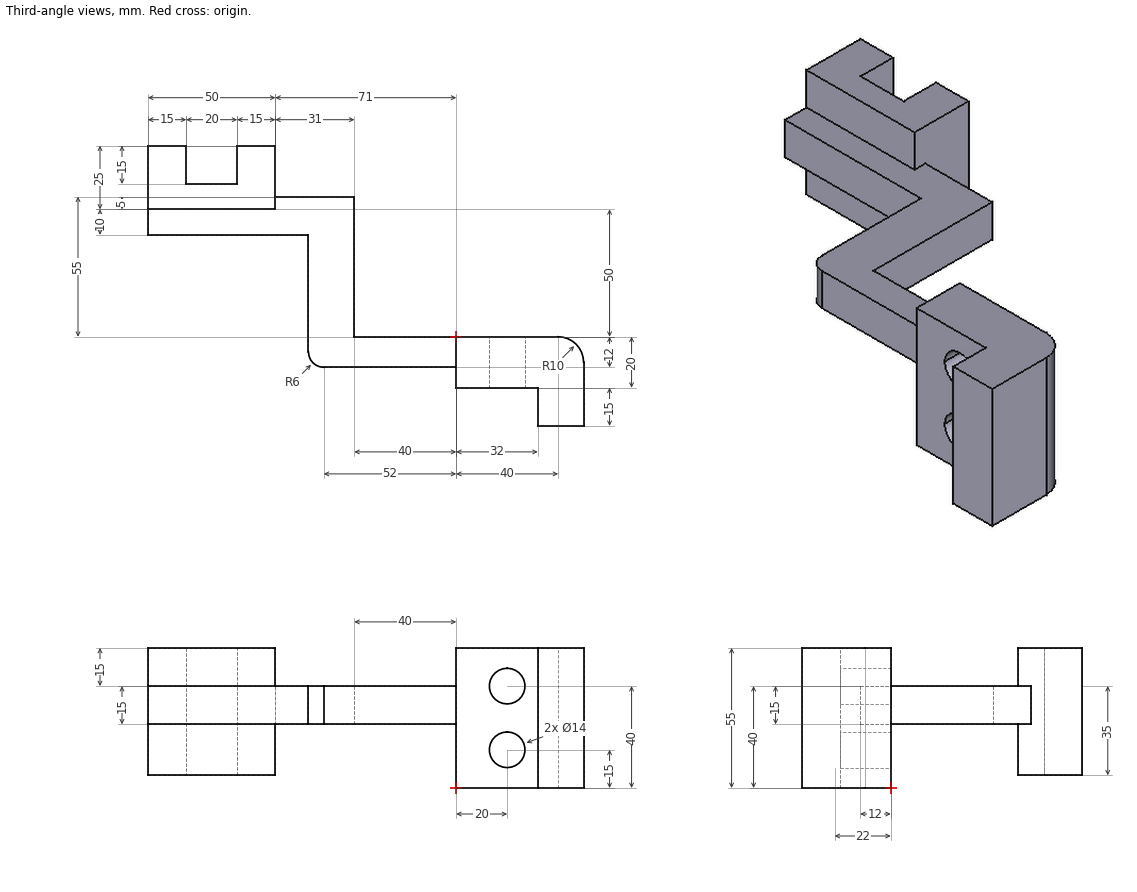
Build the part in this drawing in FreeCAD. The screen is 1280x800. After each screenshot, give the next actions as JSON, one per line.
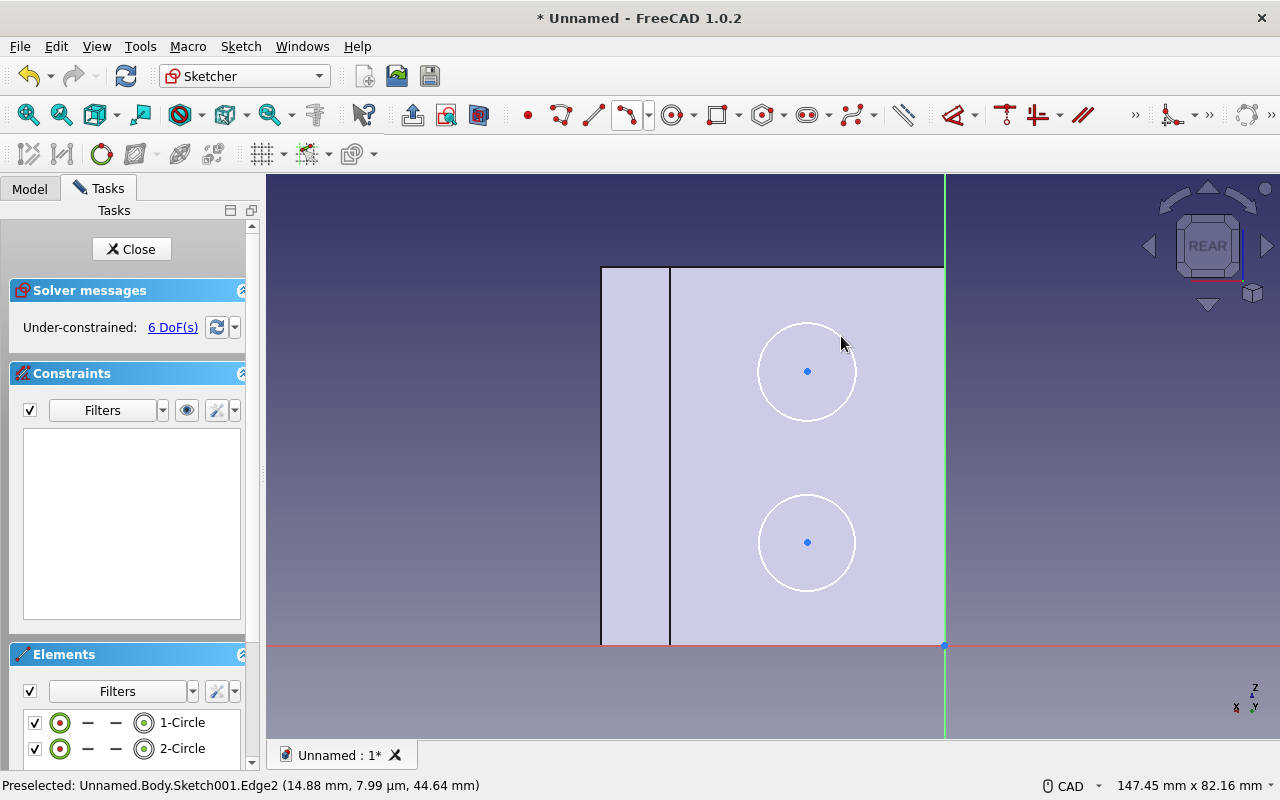
{"action": "left_click", "coordinate": [841, 509]}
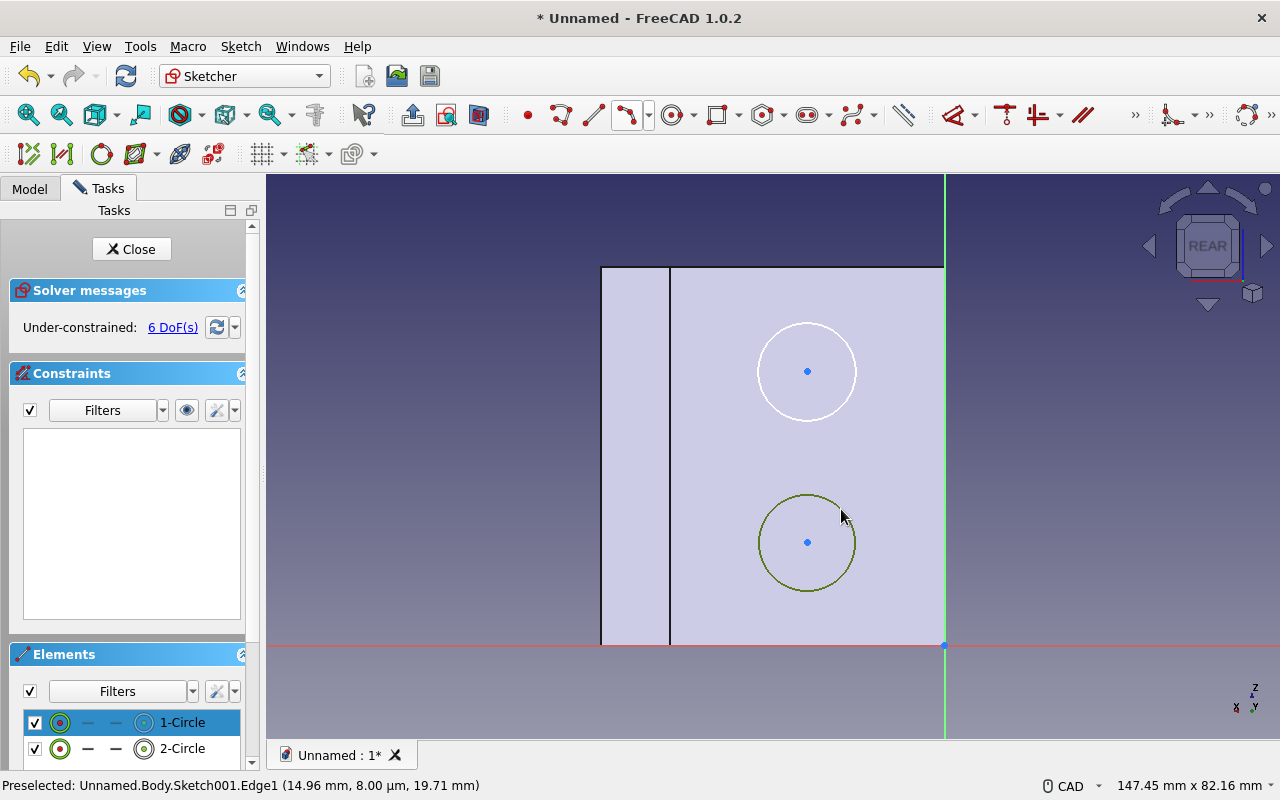
{"action": "left_click", "coordinate": [841, 337]}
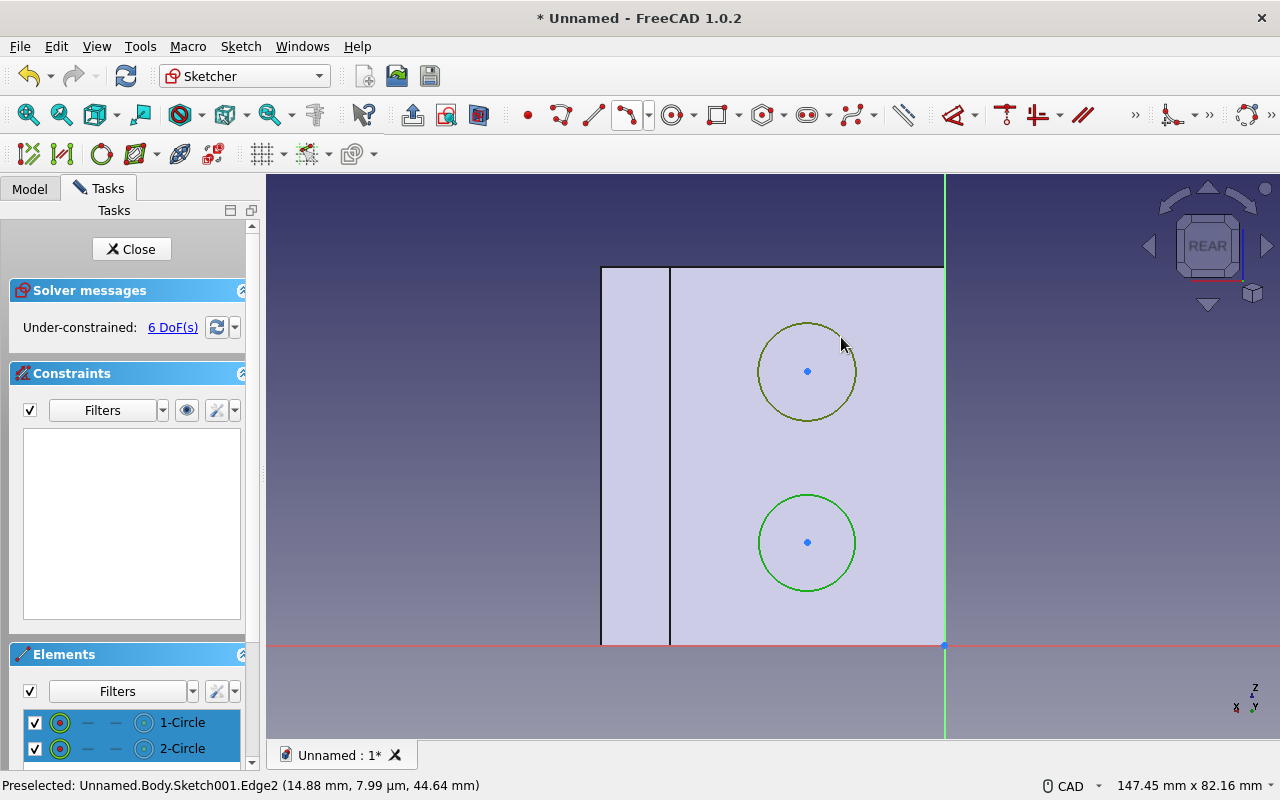
{"action": "key", "text": "e"}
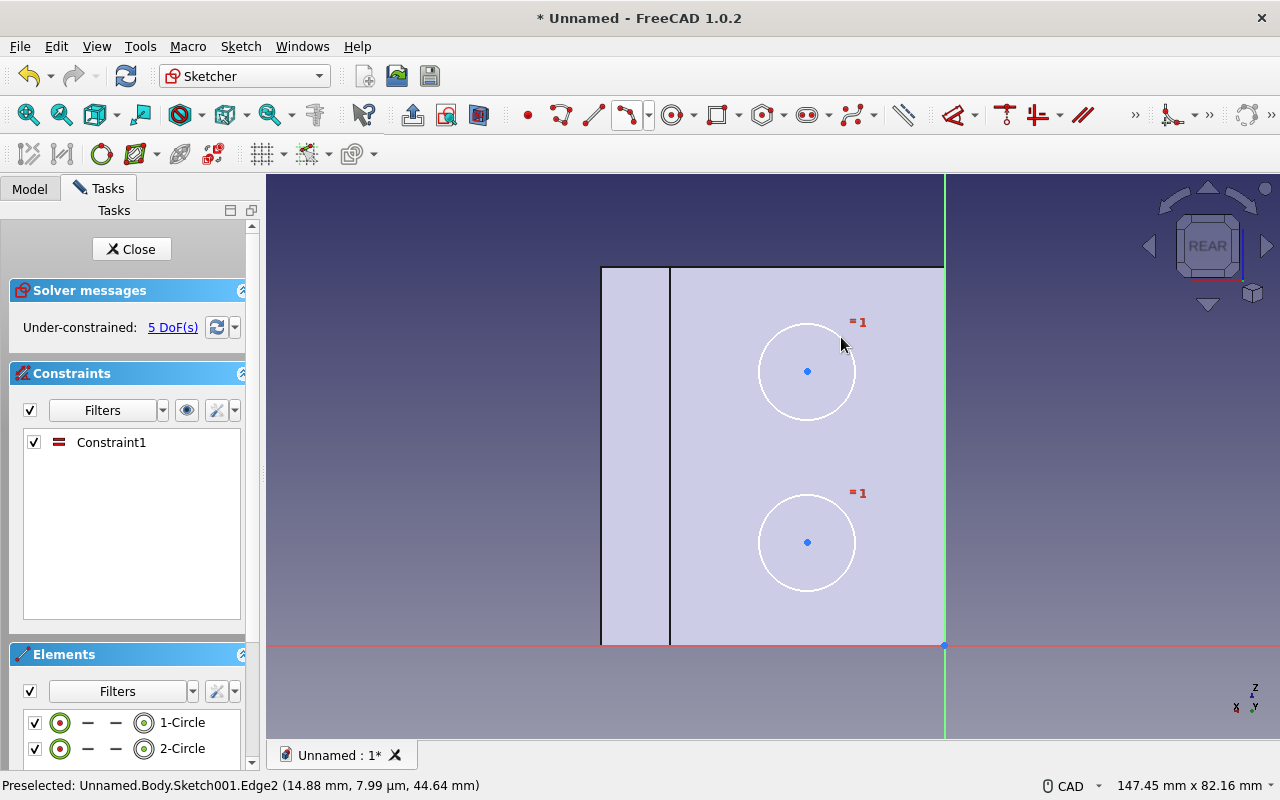
{"action": "left_click", "coordinate": [807, 543]}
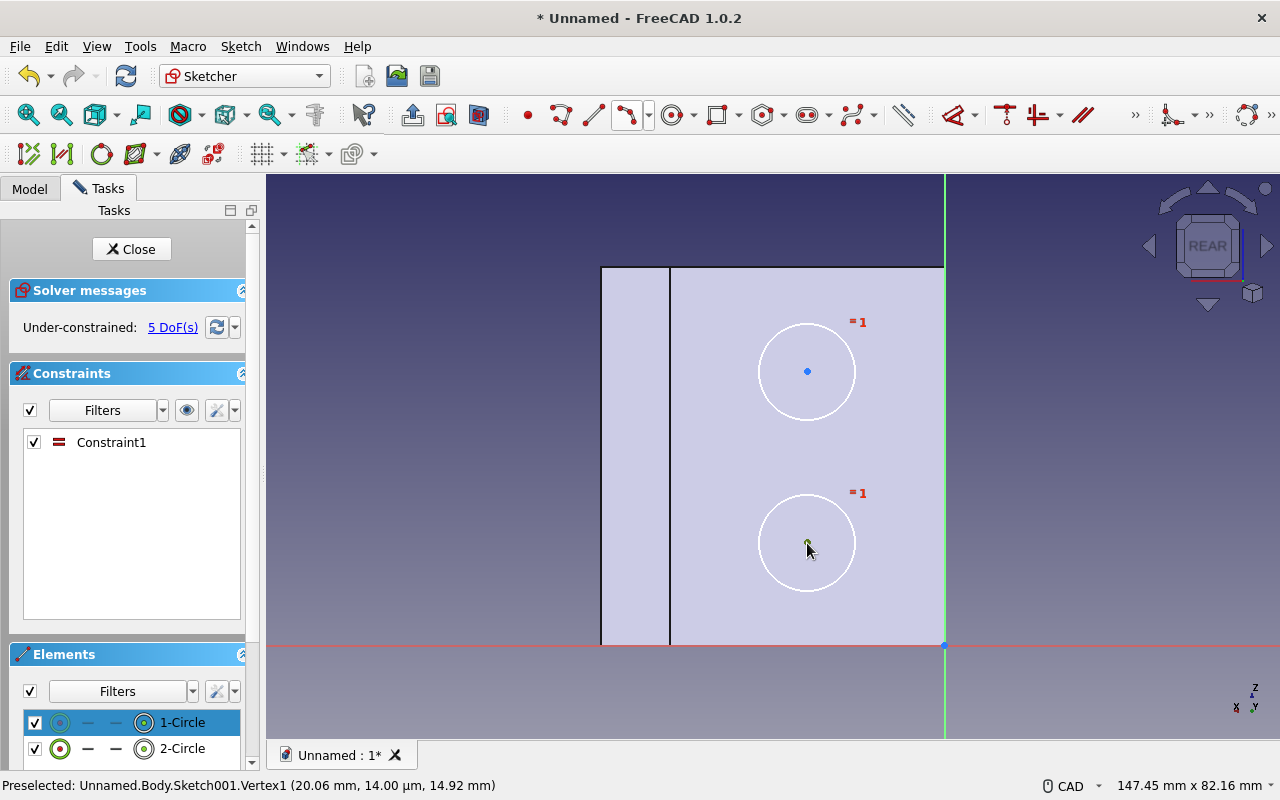
{"action": "left_click", "coordinate": [807, 372]}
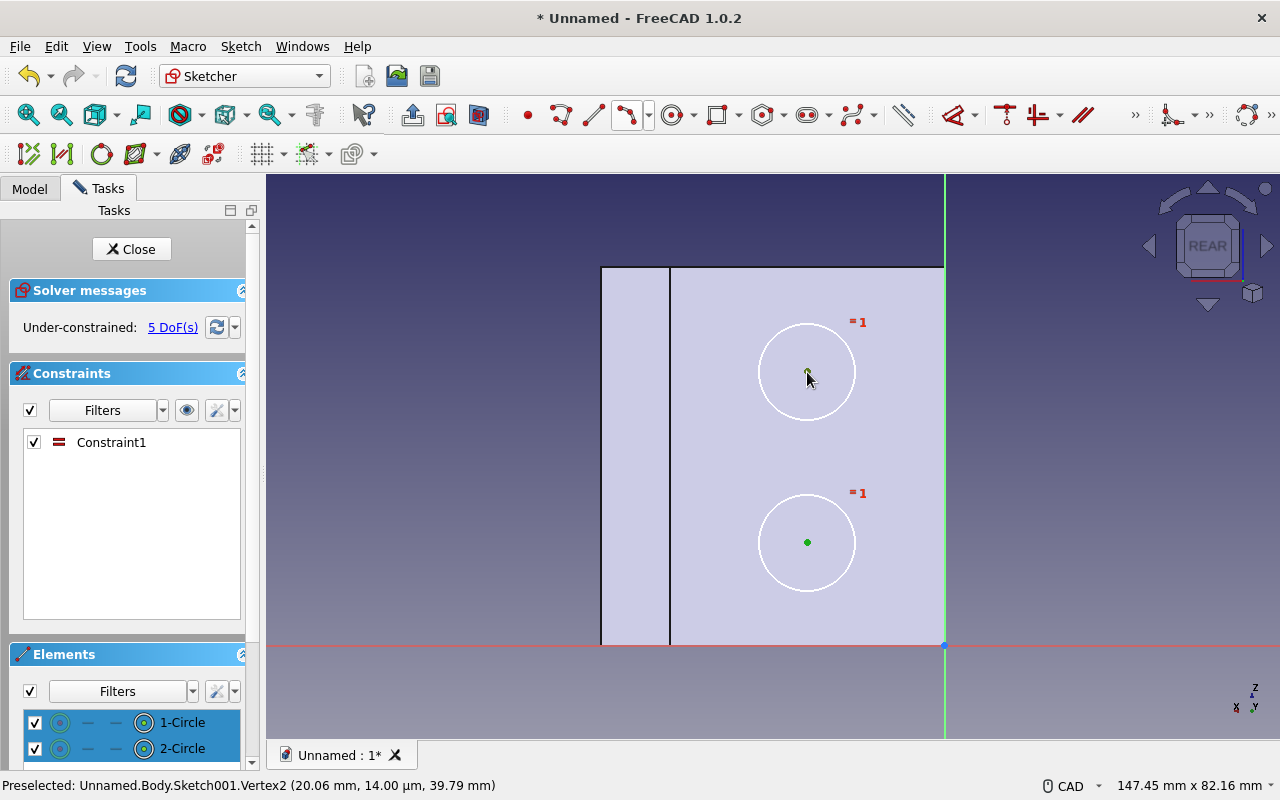
{"action": "left_click", "coordinate": [1060, 116]}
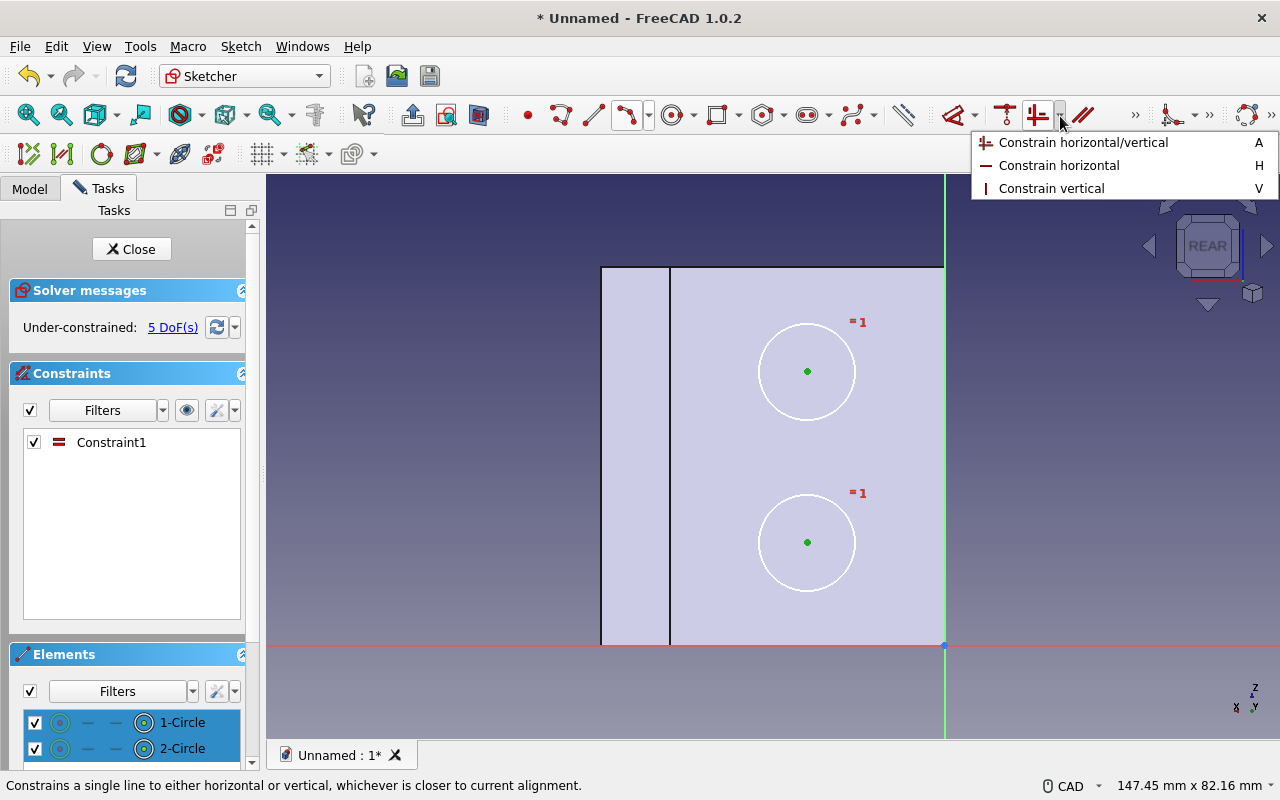
{"action": "left_click", "coordinate": [1125, 188]}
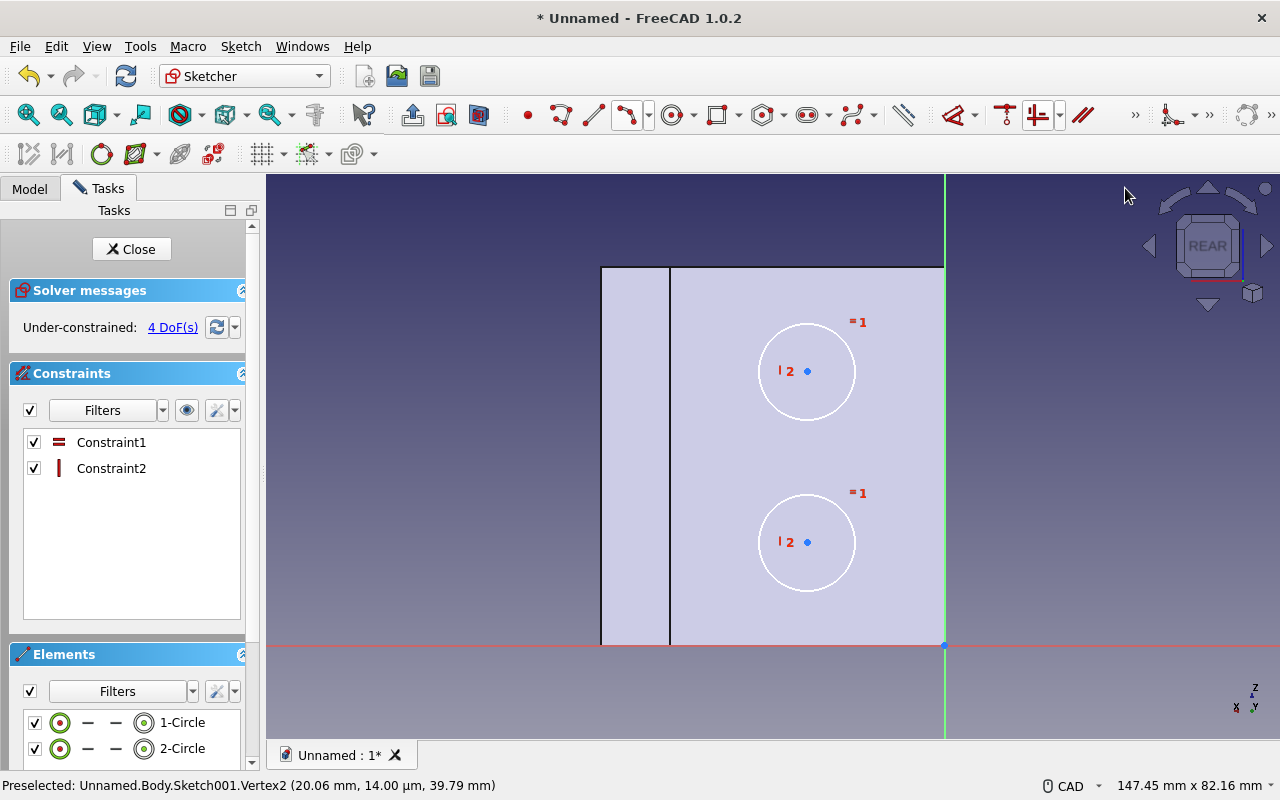
{"action": "left_click", "coordinate": [952, 116]}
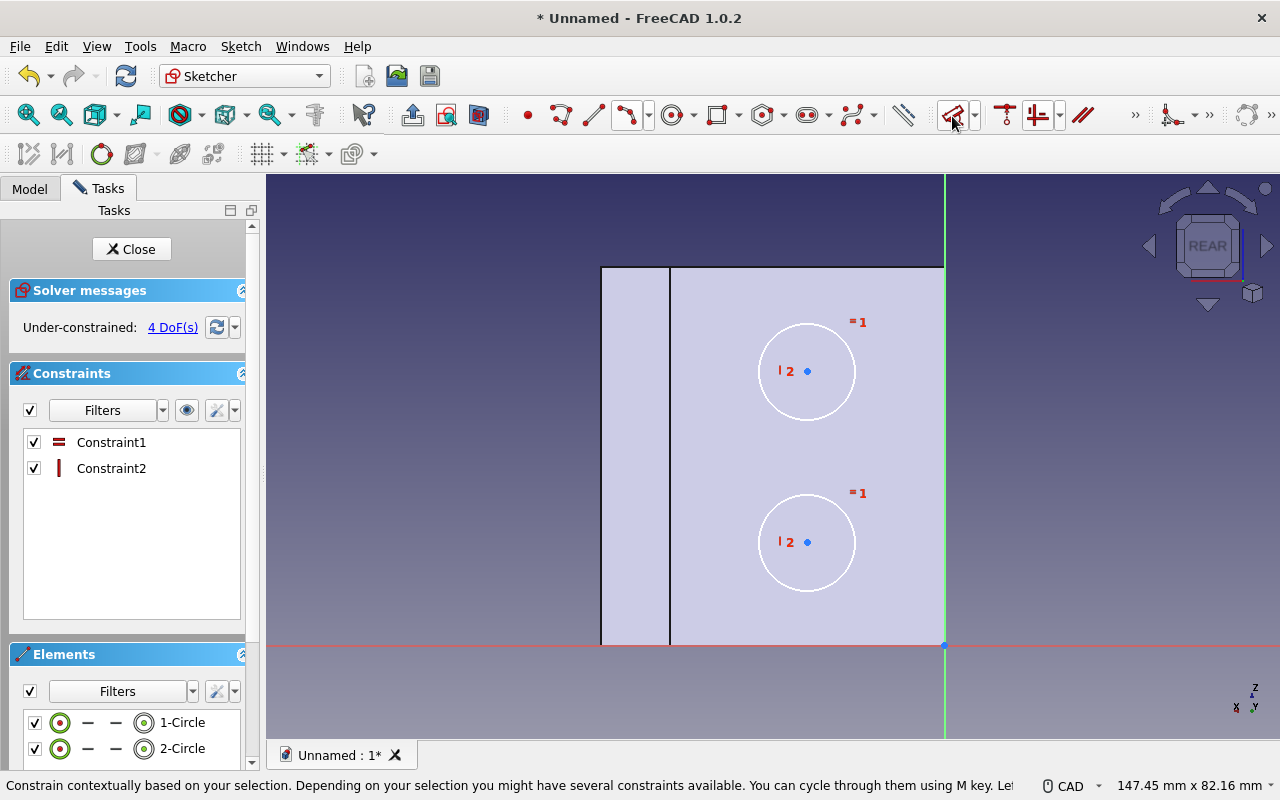
{"action": "left_click", "coordinate": [841, 509]}
{"action": "left_click", "coordinate": [864, 486]}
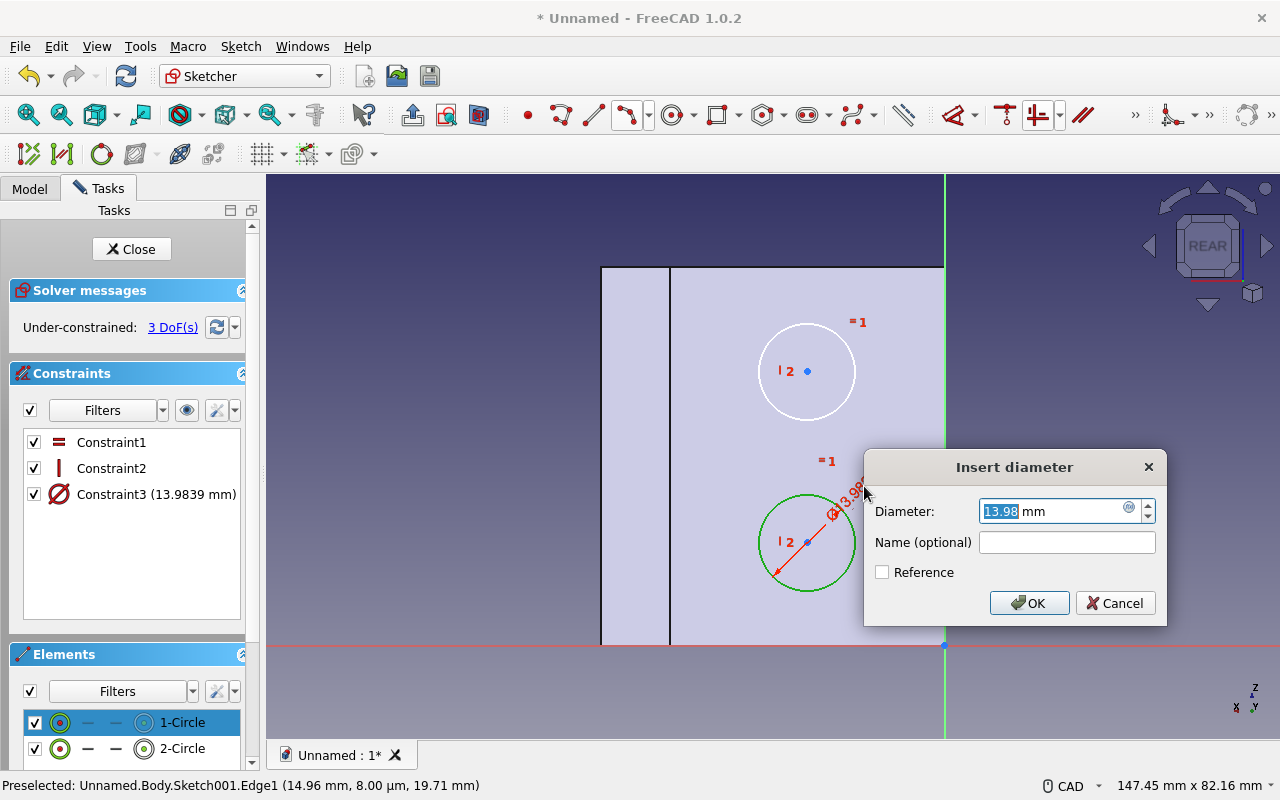
{"action": "type", "text": "14"}
{"action": "key", "text": "Return"}